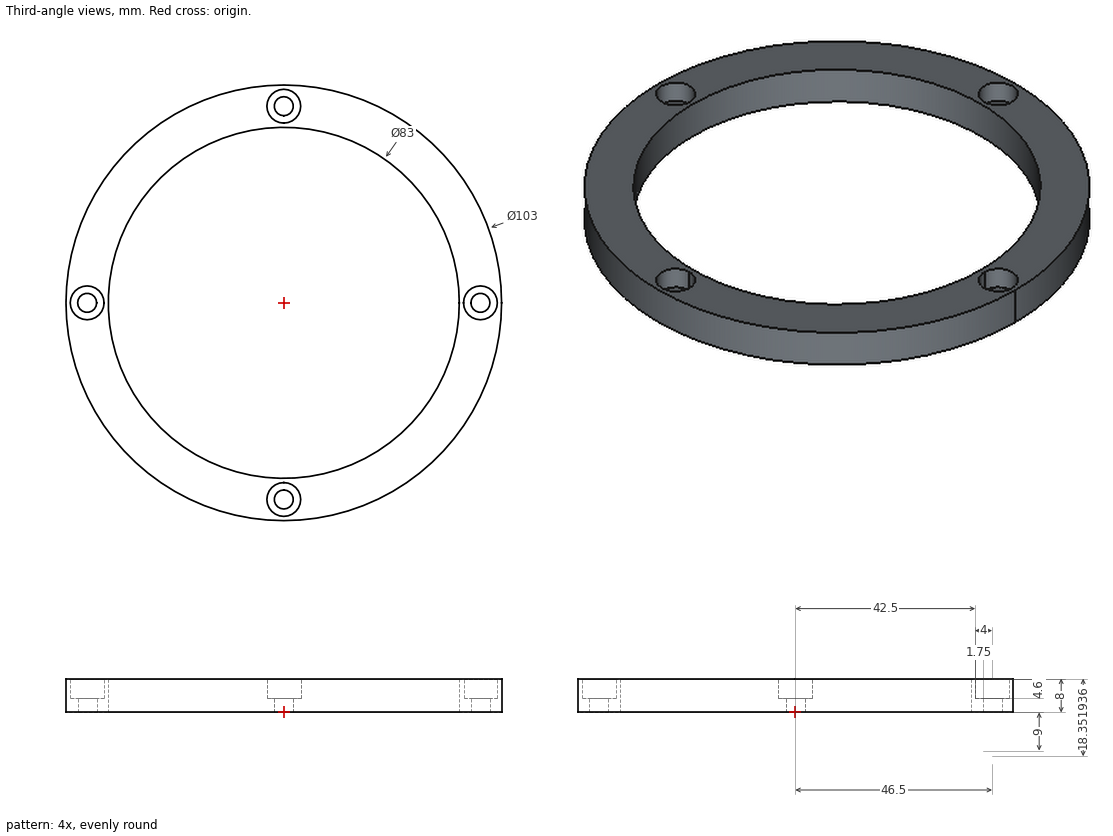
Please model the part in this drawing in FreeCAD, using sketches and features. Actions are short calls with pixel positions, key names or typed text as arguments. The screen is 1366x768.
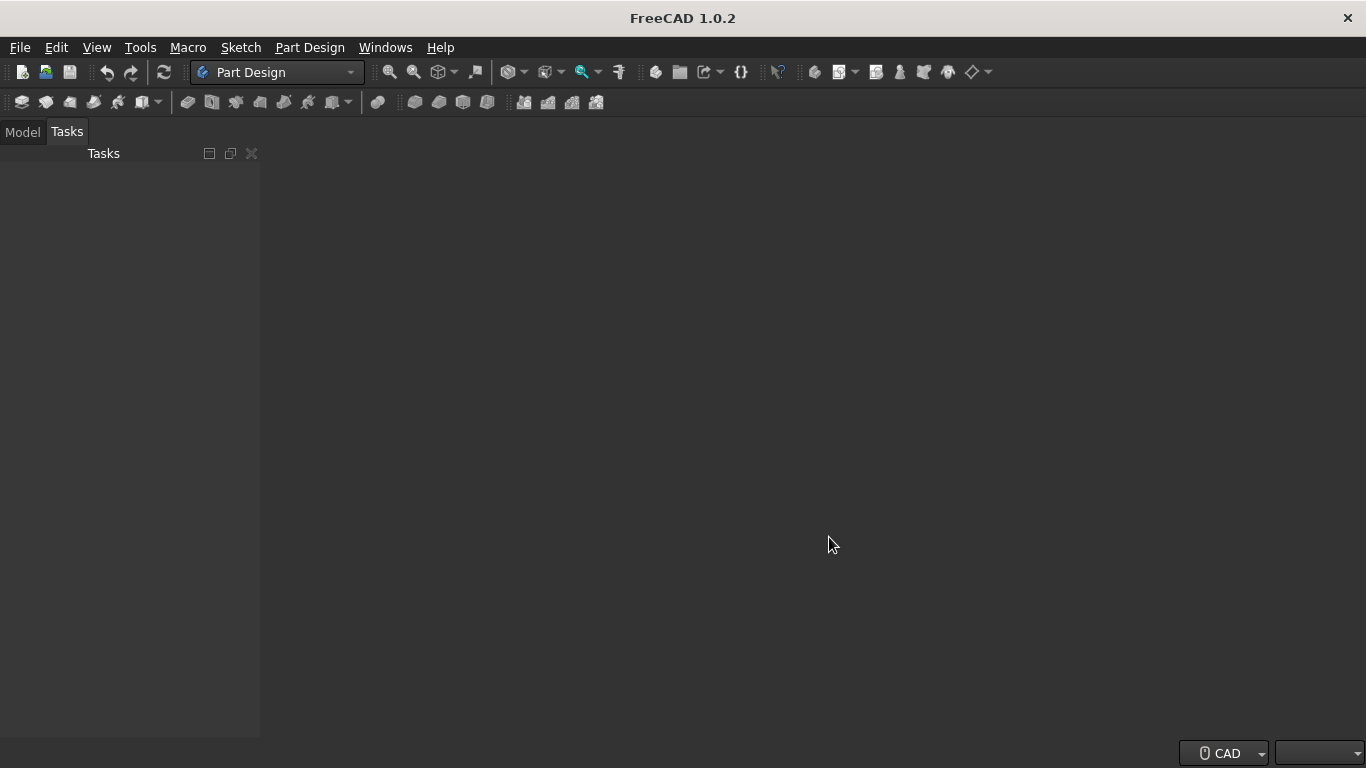
key(ctrl+n)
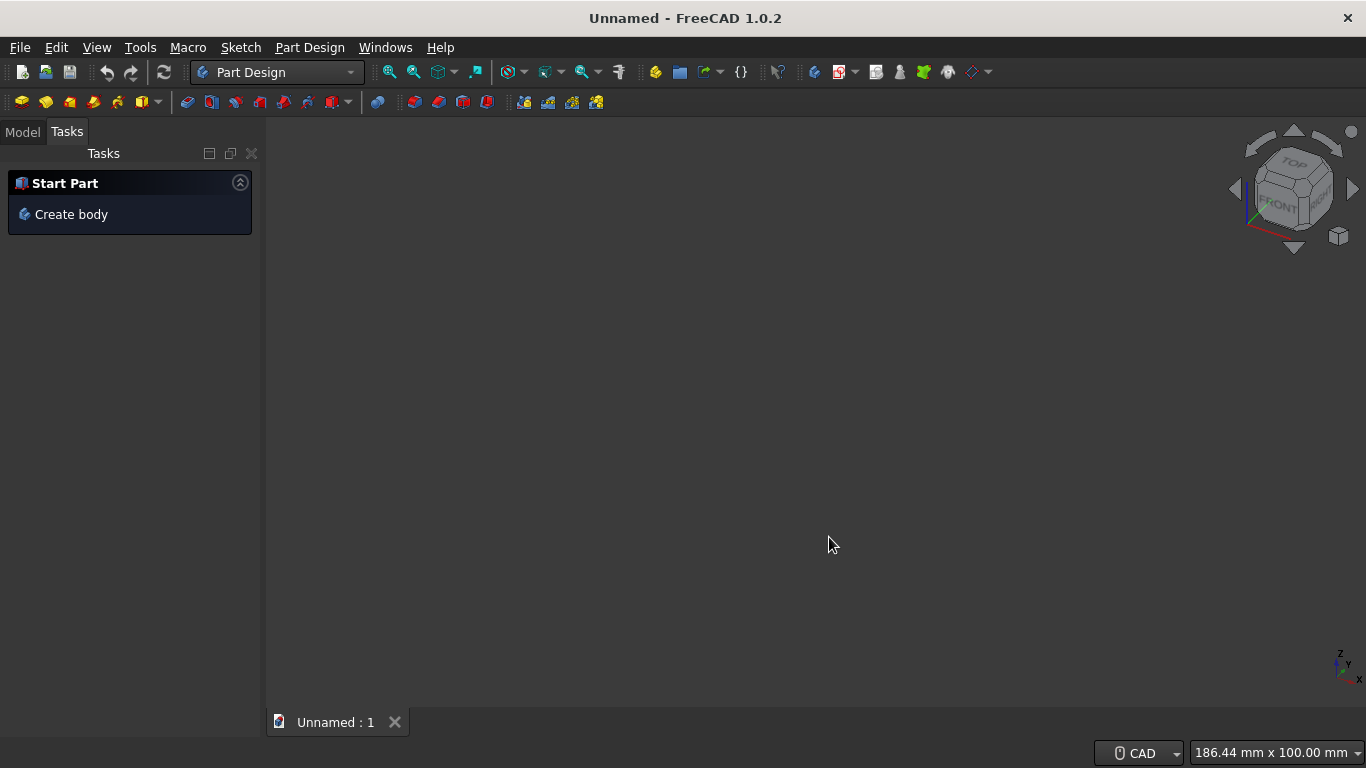
click(840, 72)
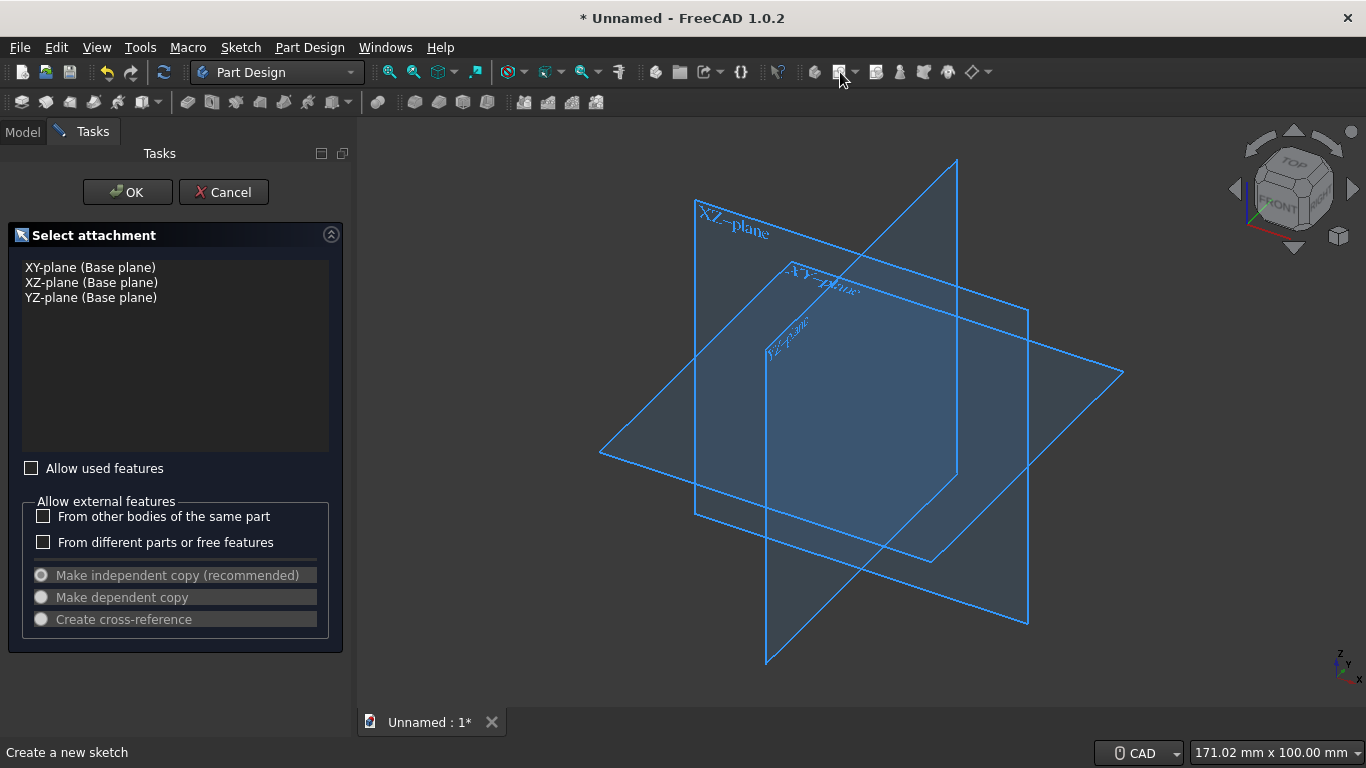
click(82, 268)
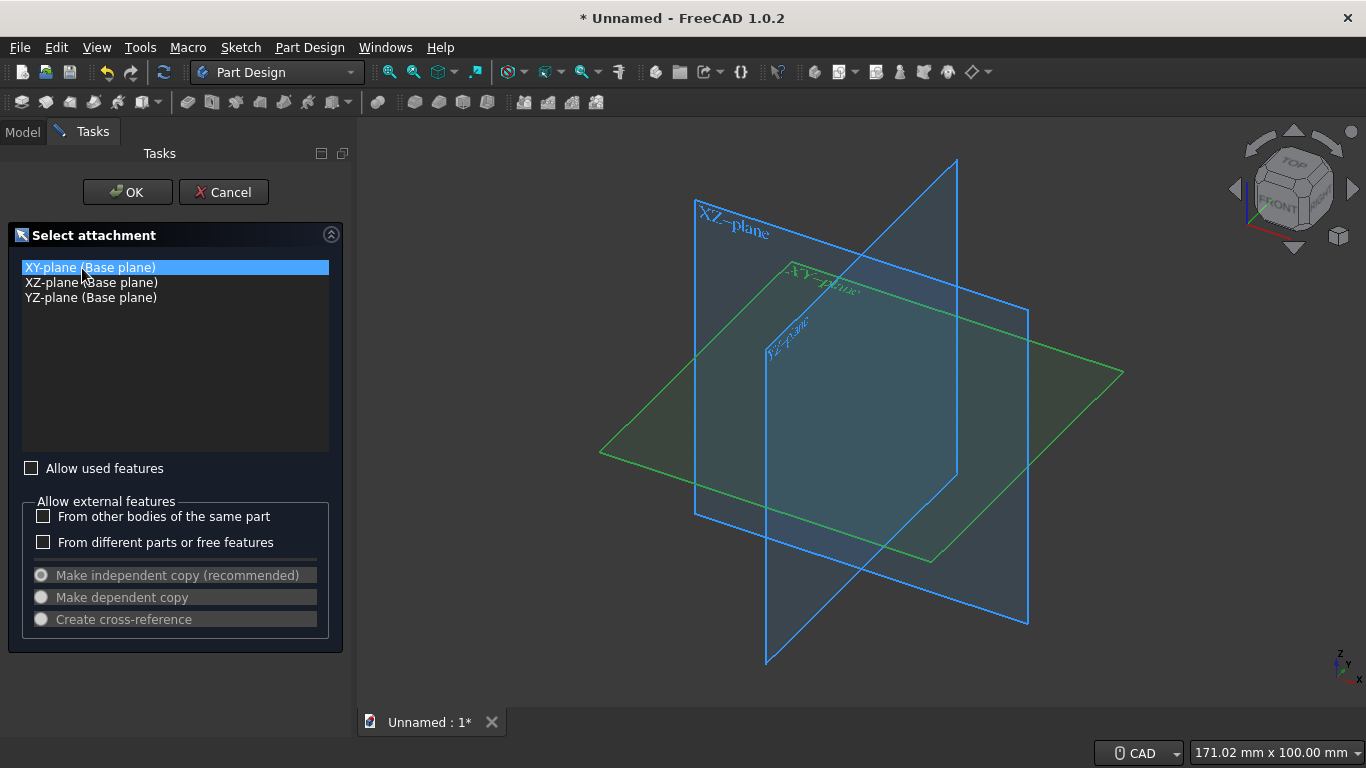
click(128, 192)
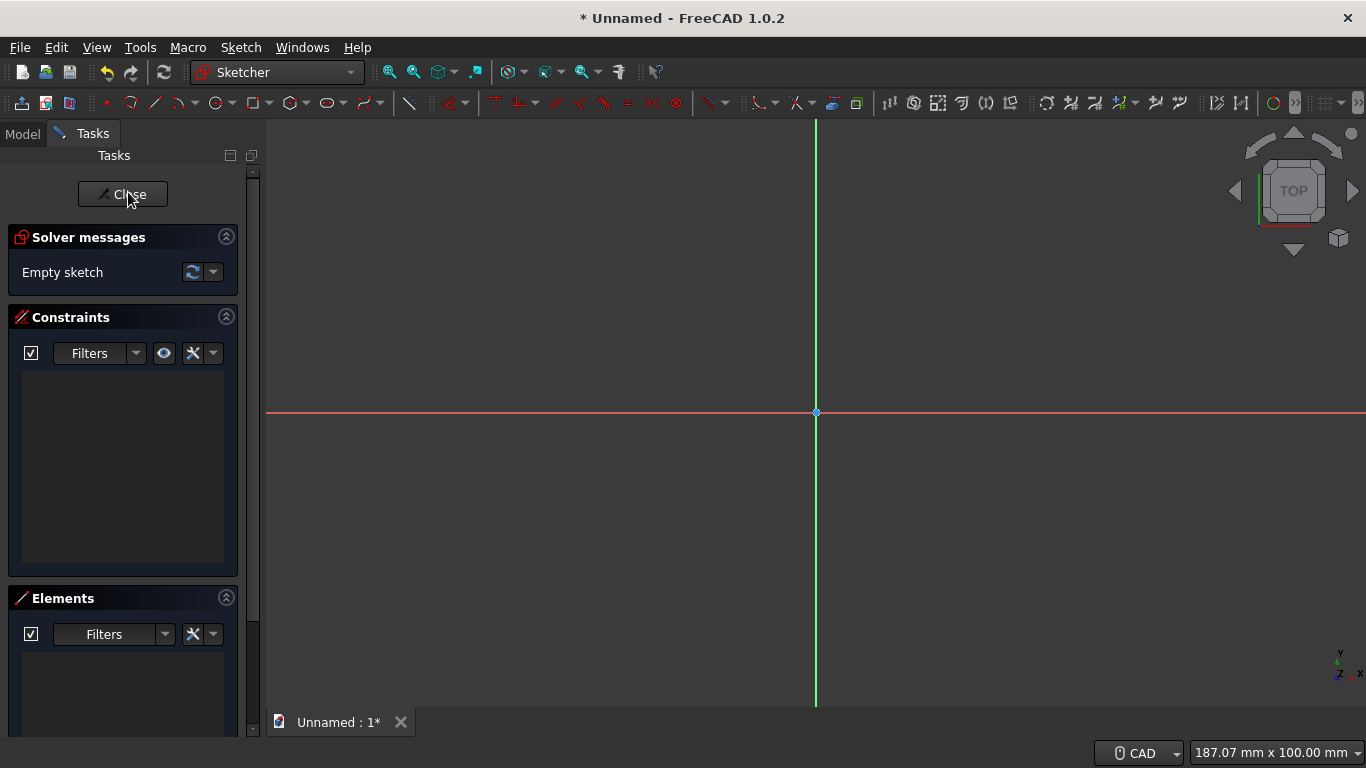
scroll(608, 413, down, 2)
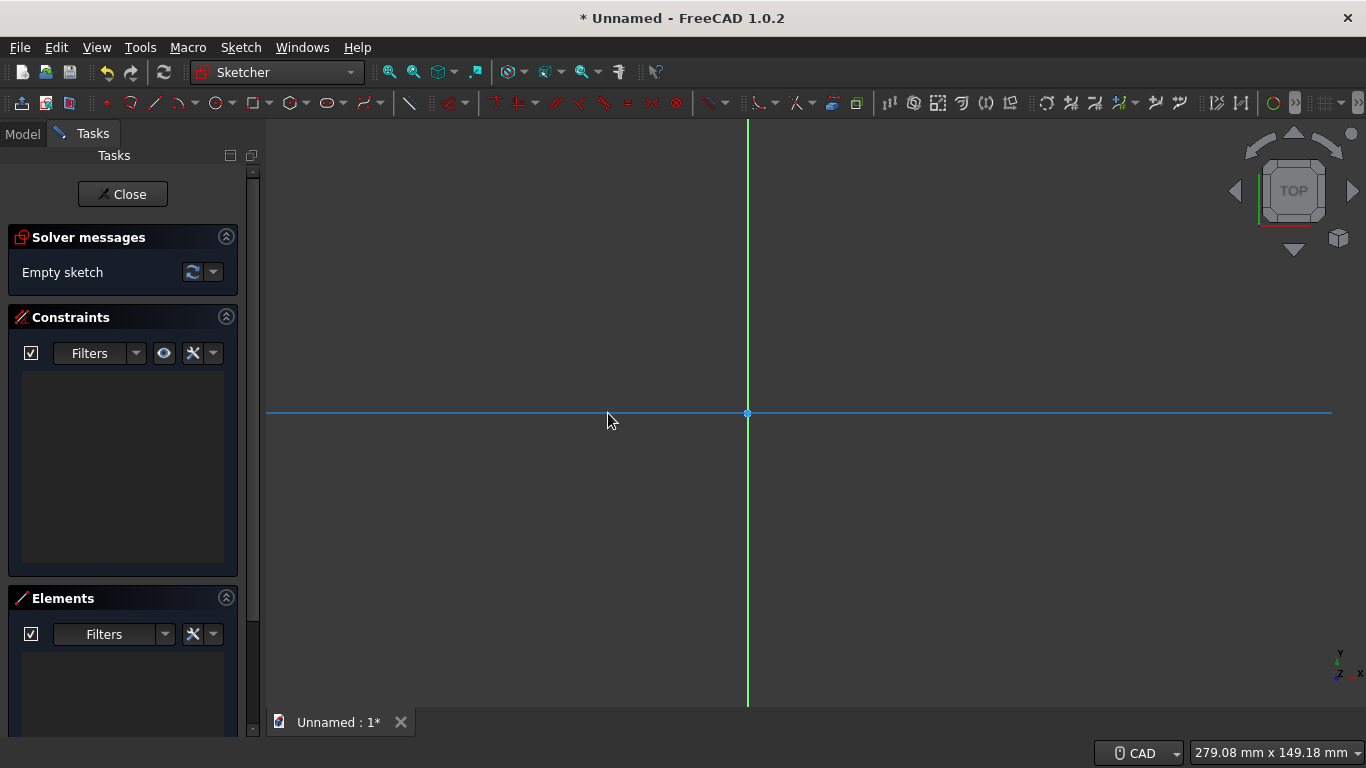
click(216, 104)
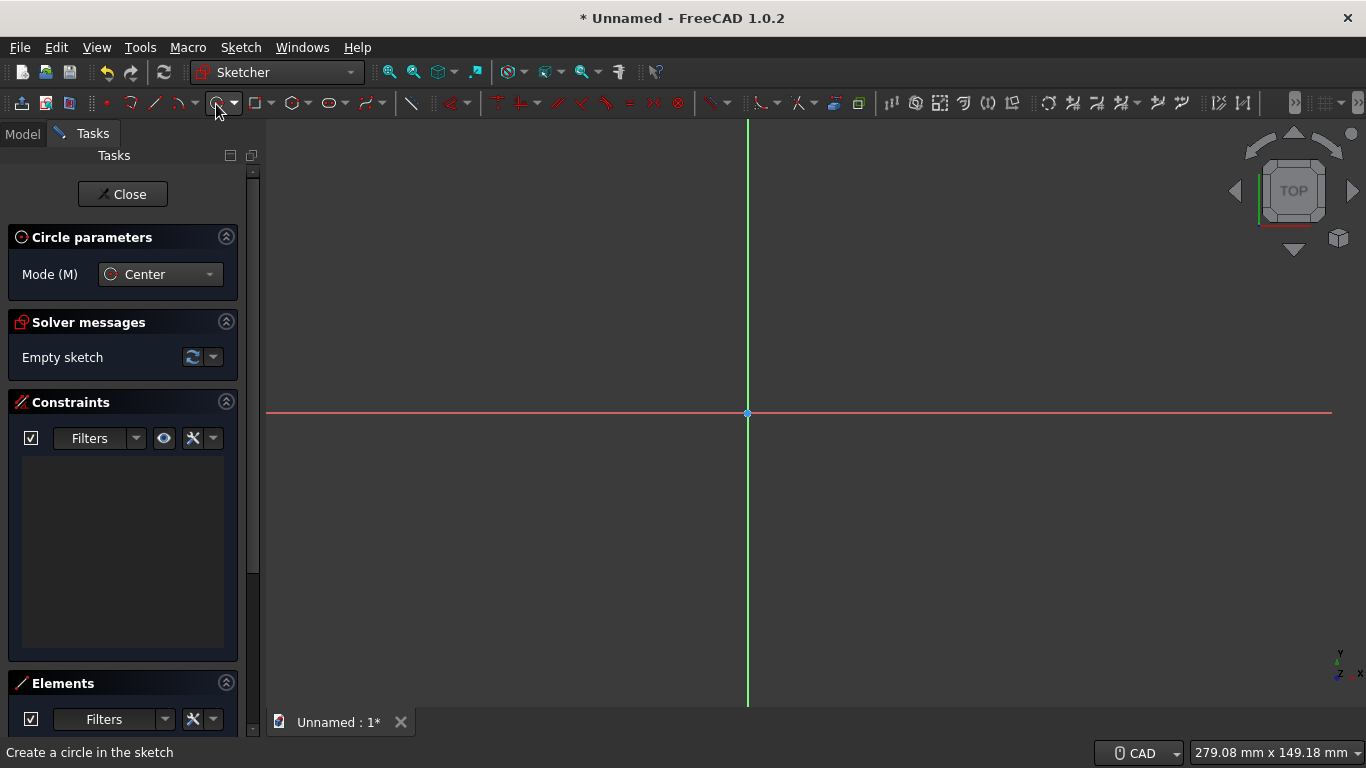
click(748, 413)
move(891, 270)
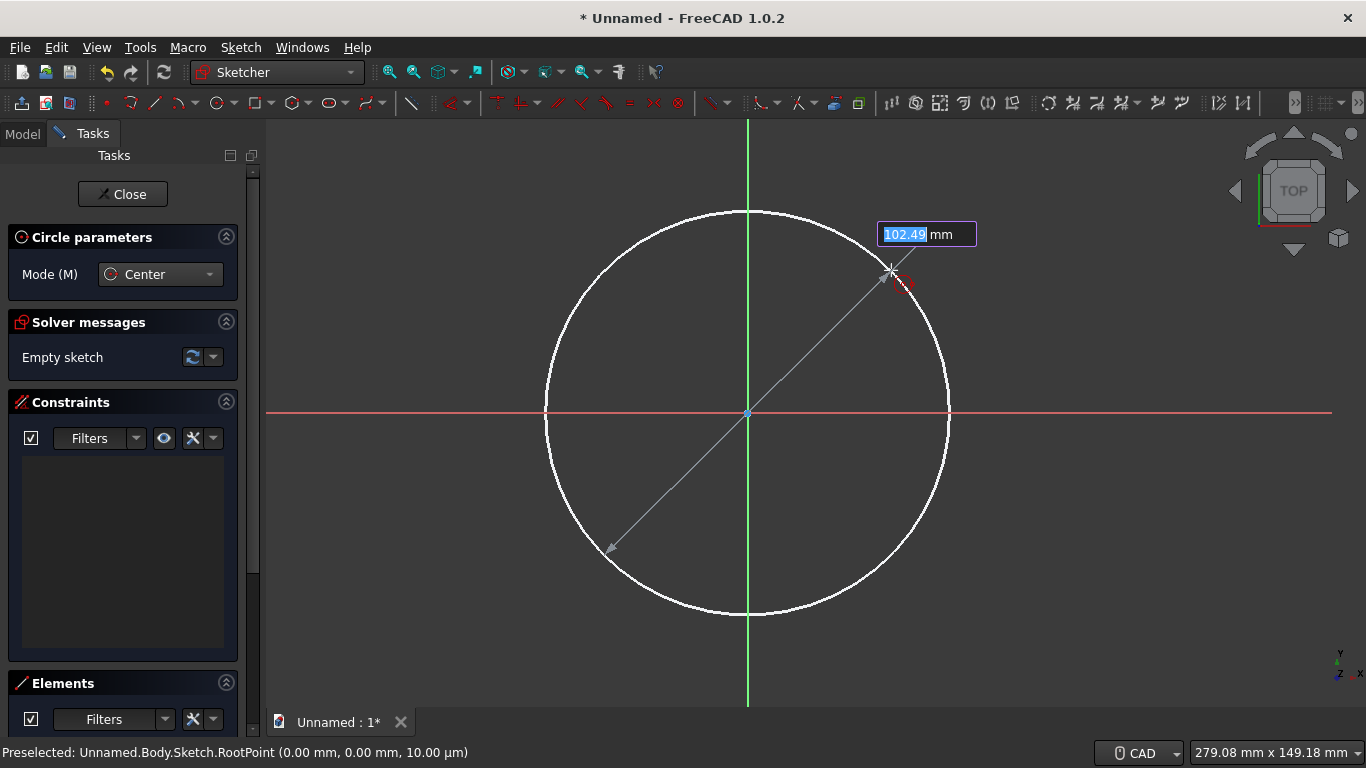
text(103)
key(Return)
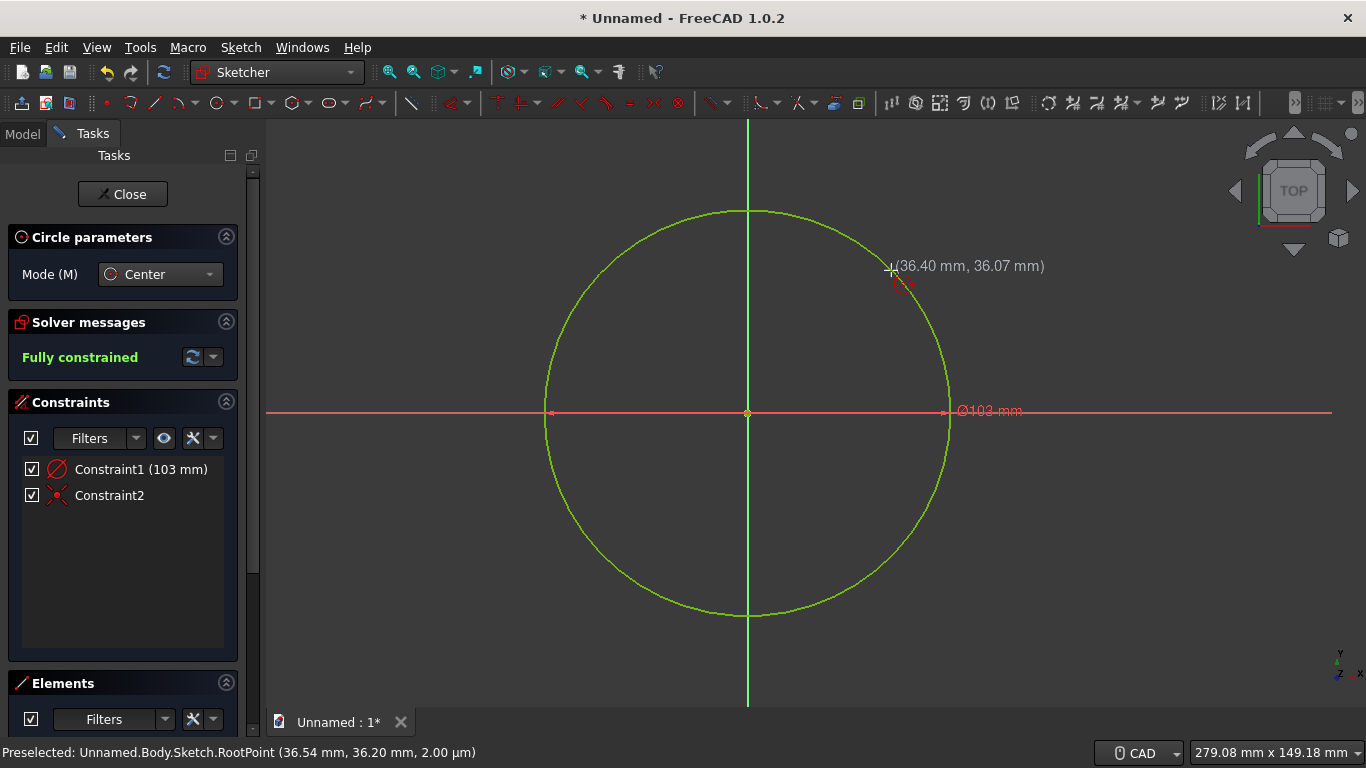
click(748, 413)
move(863, 298)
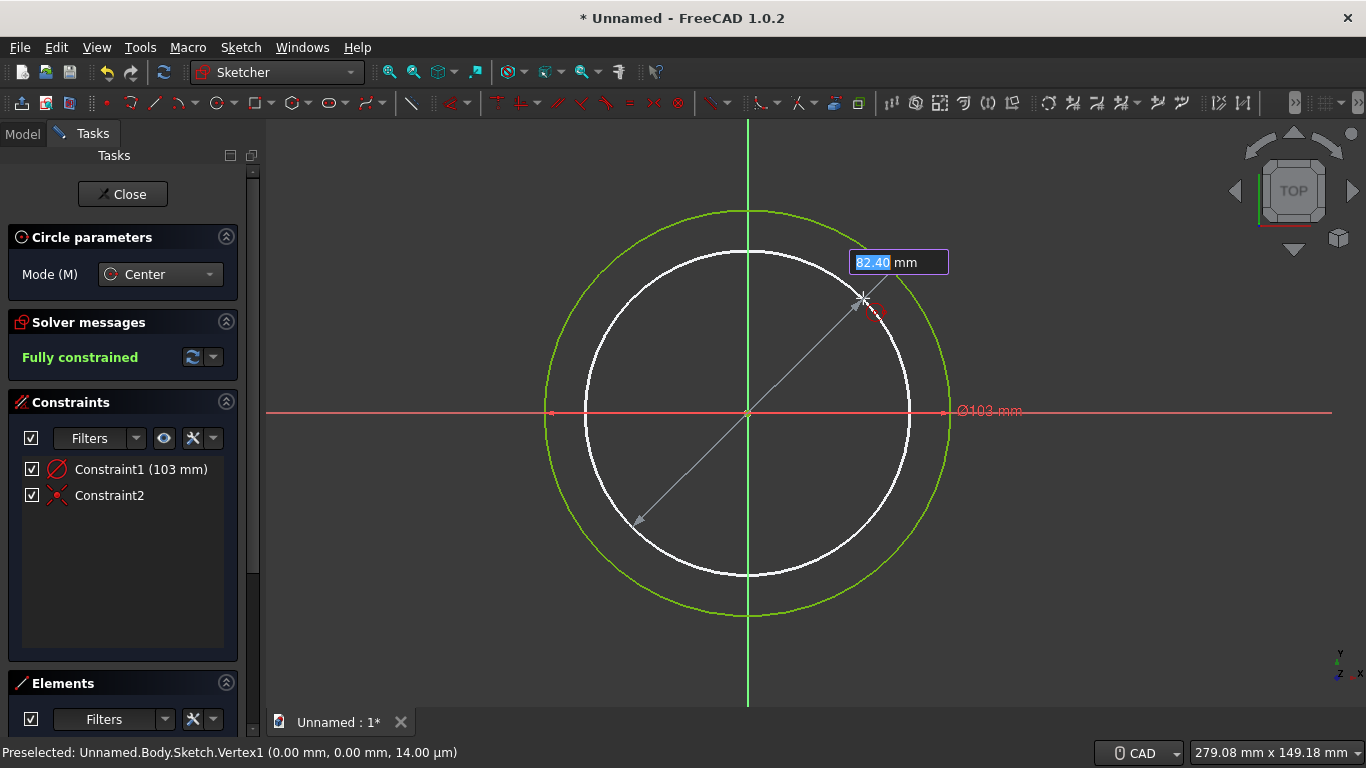
text(83)
key(Return)
key(Escape)